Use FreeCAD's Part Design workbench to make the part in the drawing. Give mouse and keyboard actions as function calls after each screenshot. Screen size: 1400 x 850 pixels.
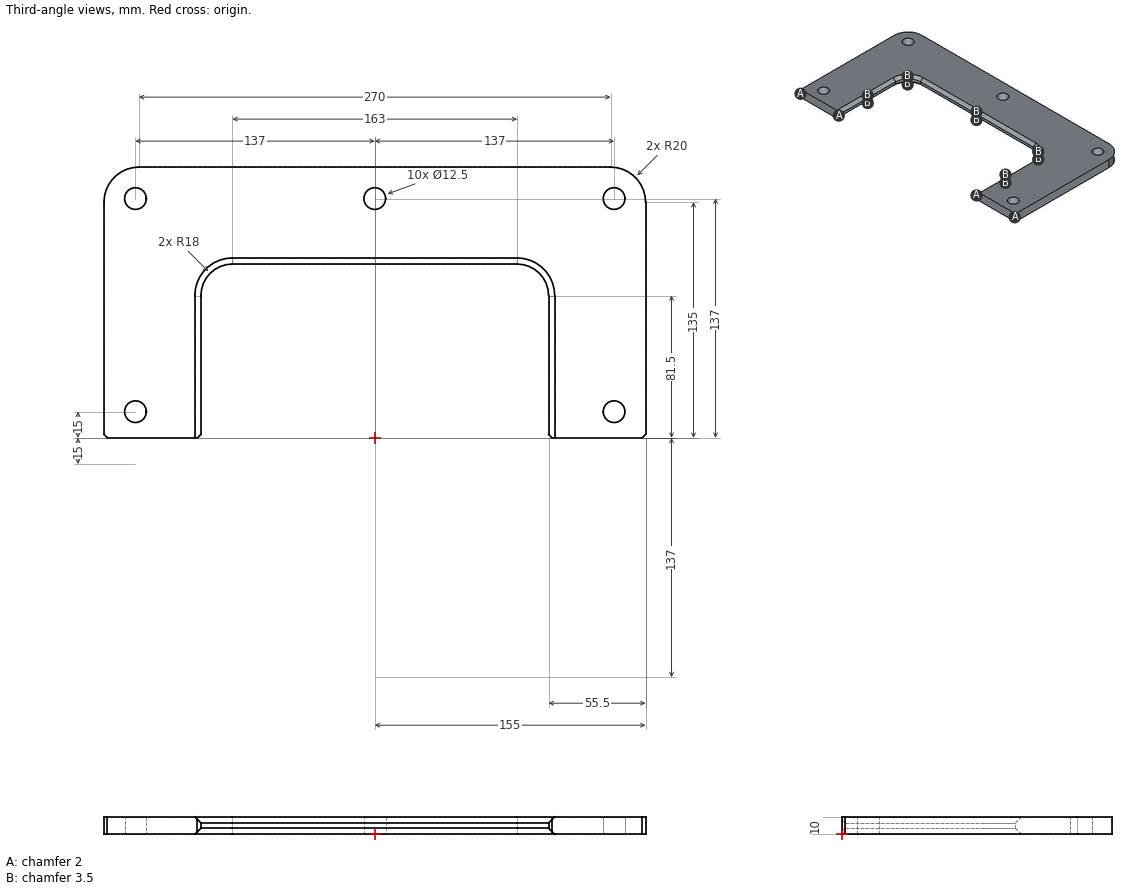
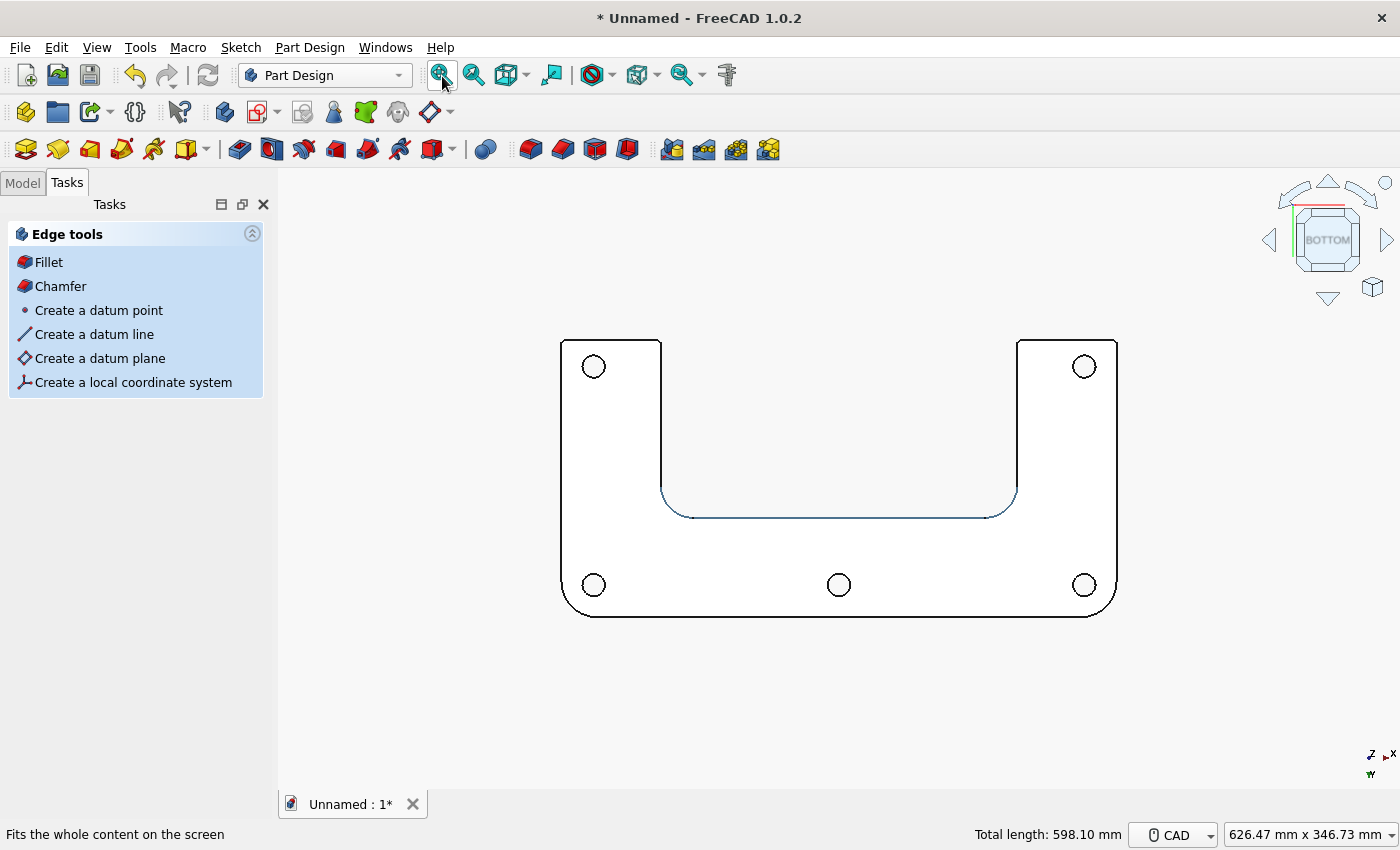
click(1017, 413, ctrl)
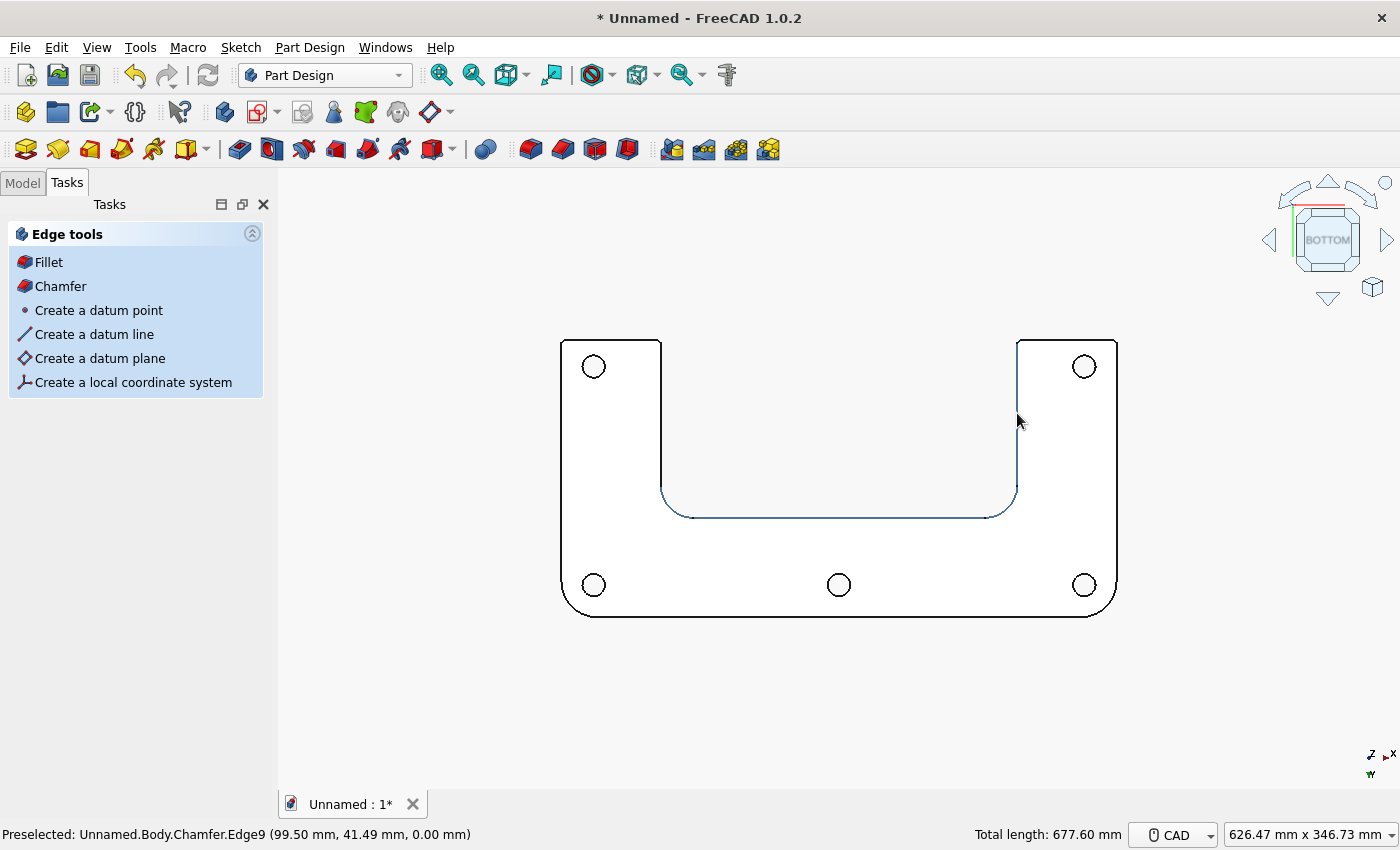
click(661, 413, ctrl)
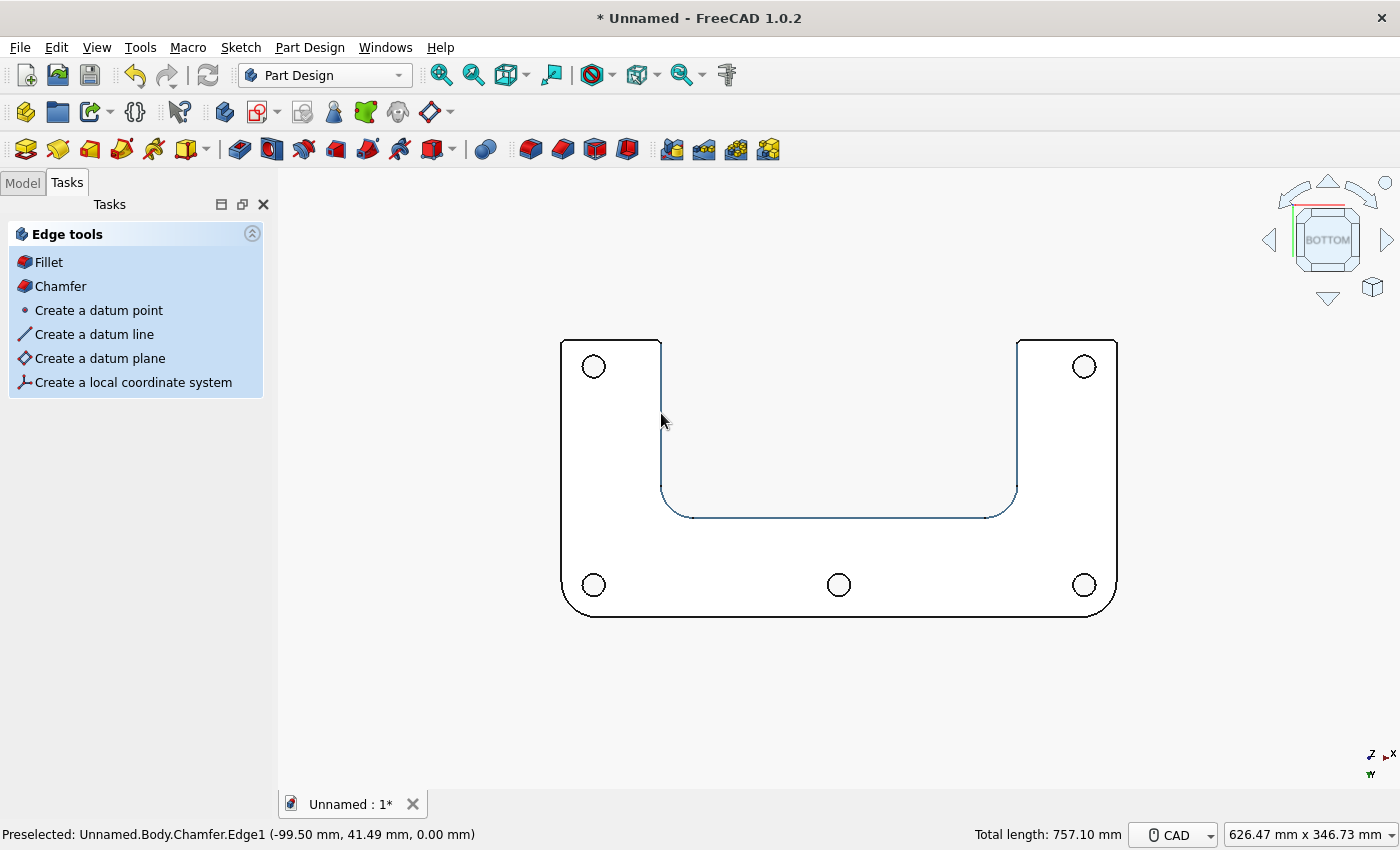
click(564, 150)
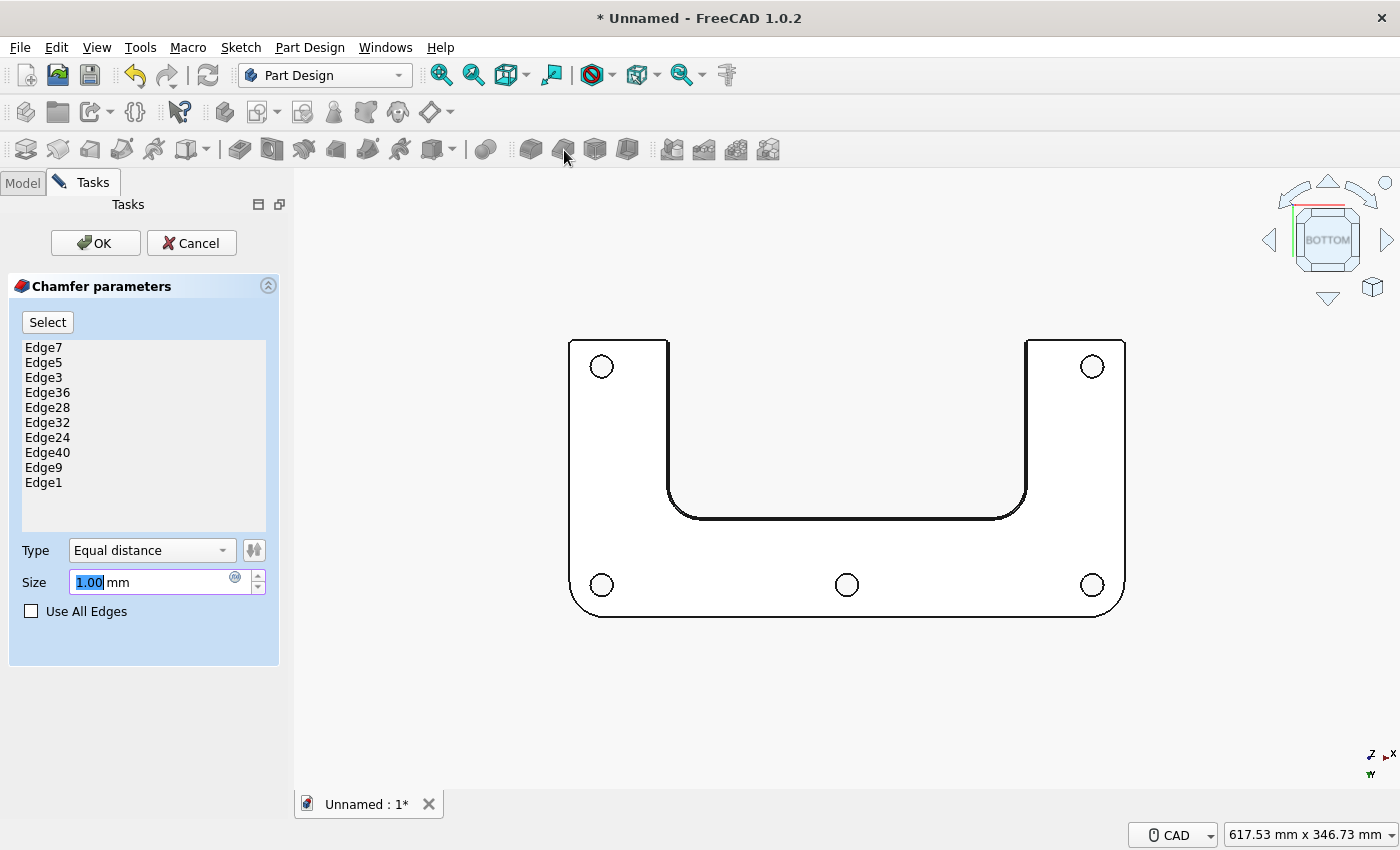
text(3.5)
key(Tab)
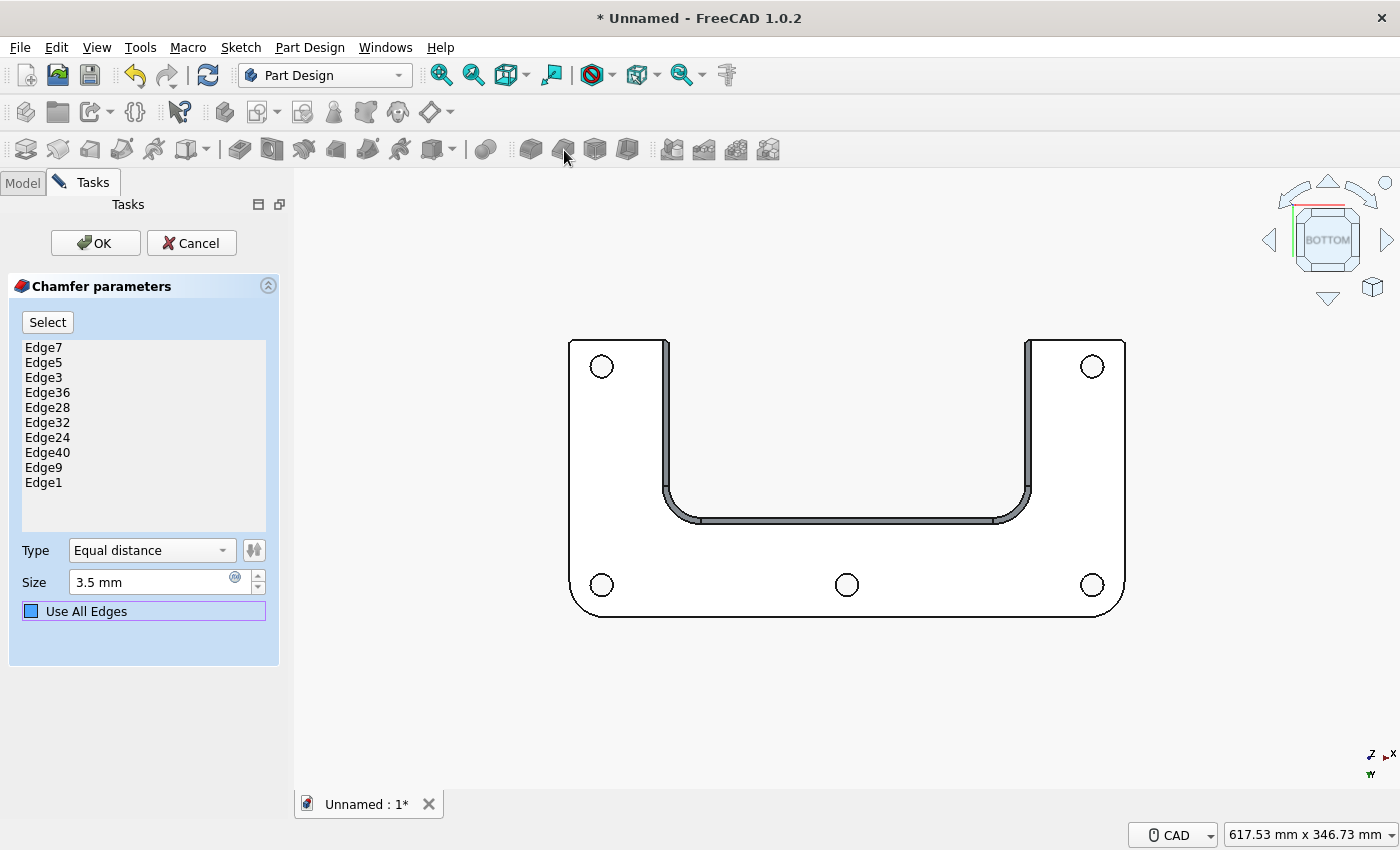
click(96, 243)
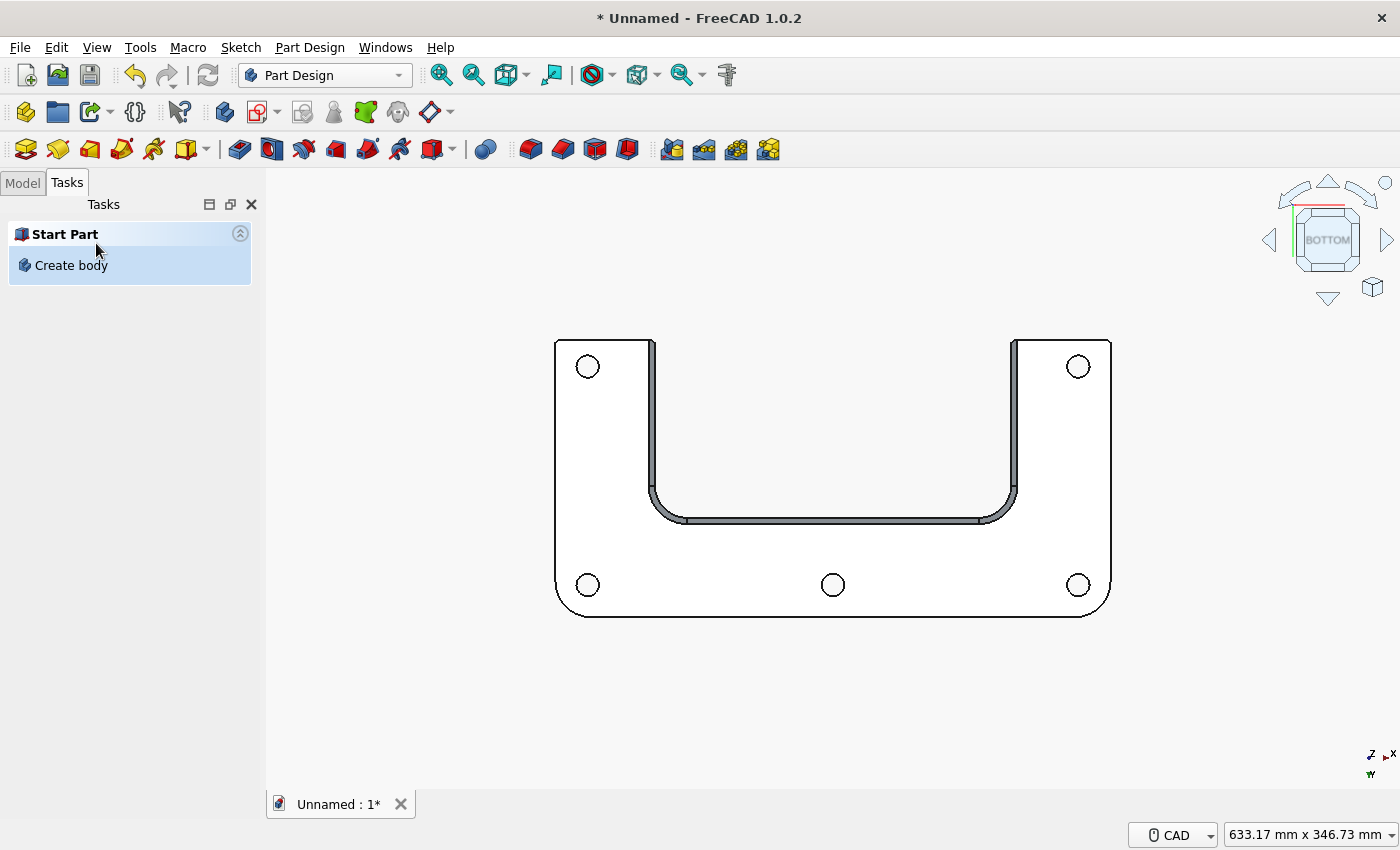
key(0)